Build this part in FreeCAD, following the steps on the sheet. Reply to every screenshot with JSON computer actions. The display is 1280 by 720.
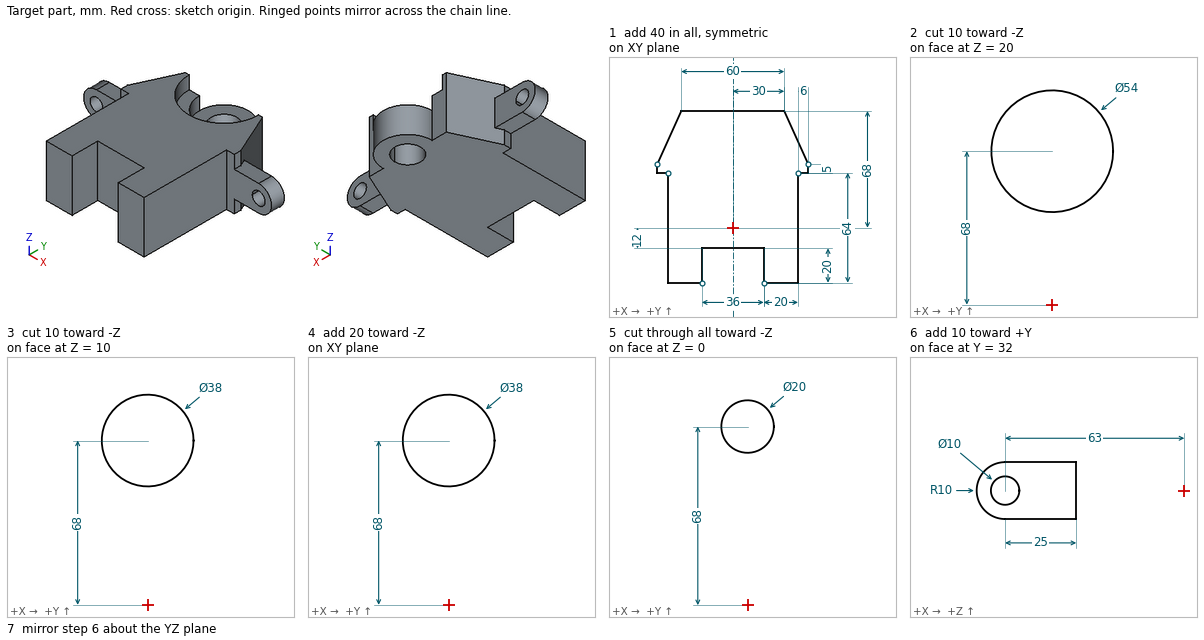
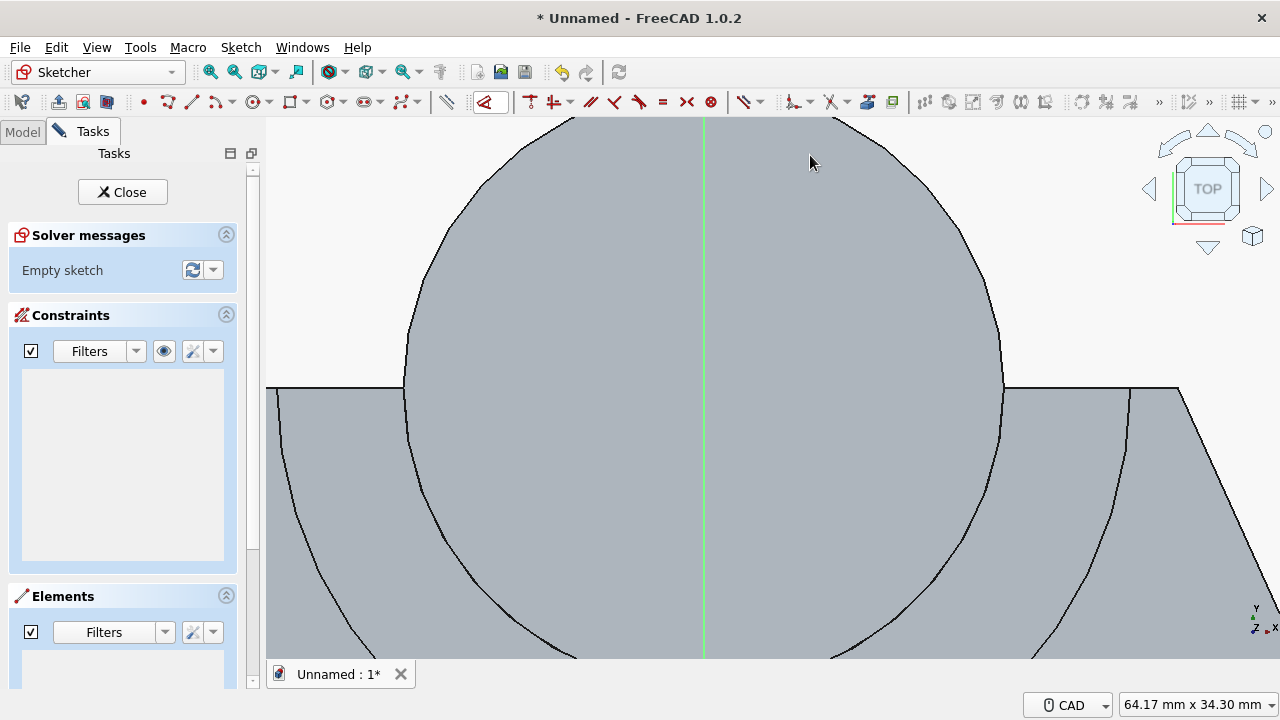
{"action": "left_click", "coordinate": [254, 102]}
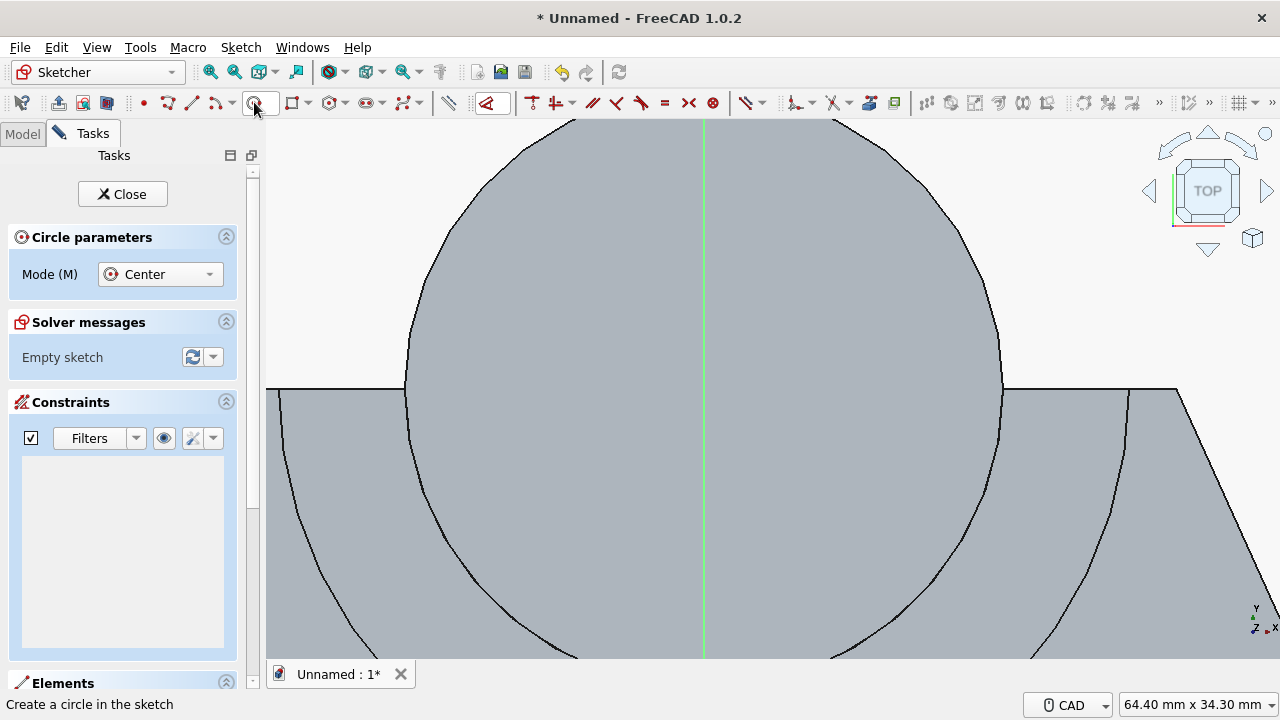
{"action": "left_click", "coordinate": [704, 389]}
{"action": "left_click", "coordinate": [815, 278]}
{"action": "key", "text": "Escape"}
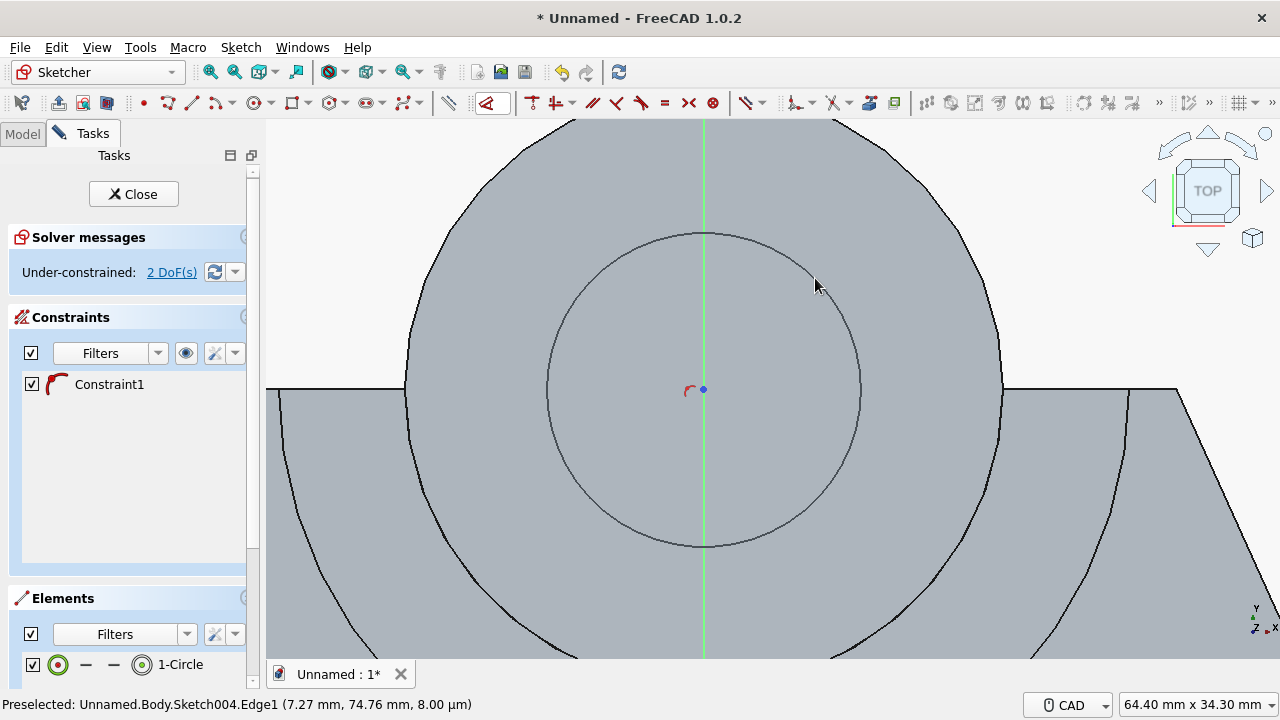
{"action": "left_click", "coordinate": [815, 279]}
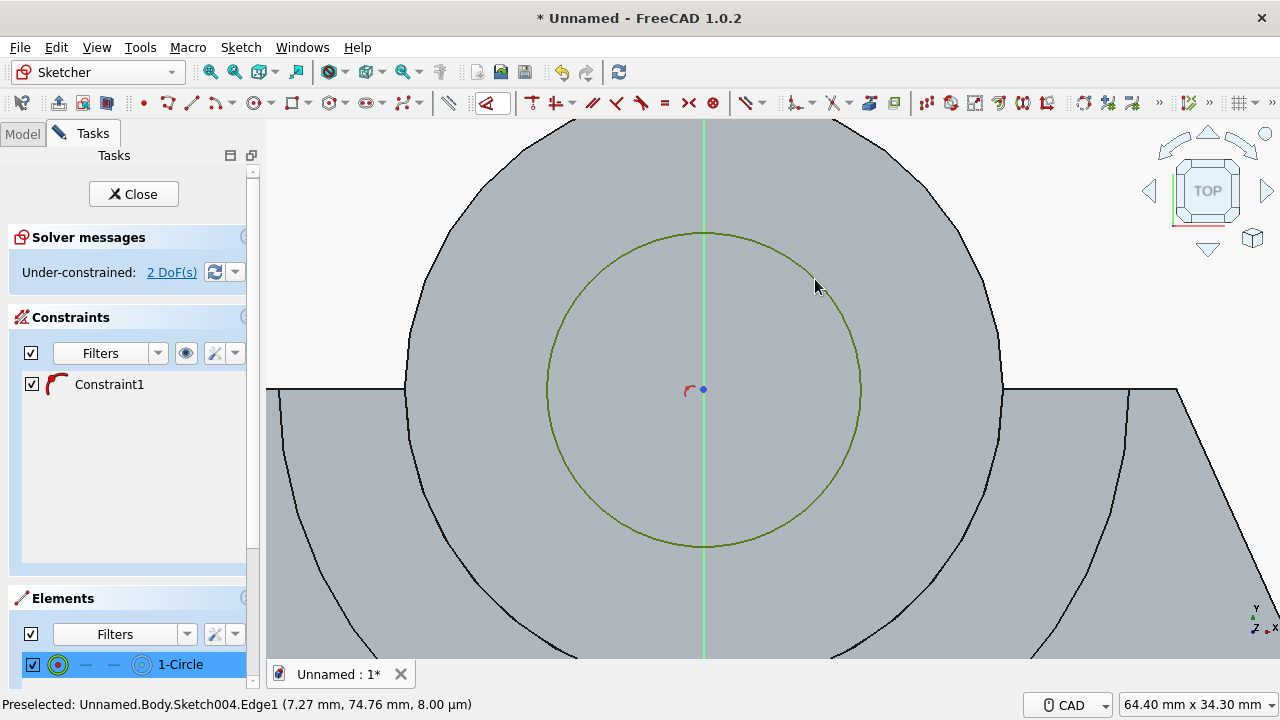
{"action": "key", "text": "k o"}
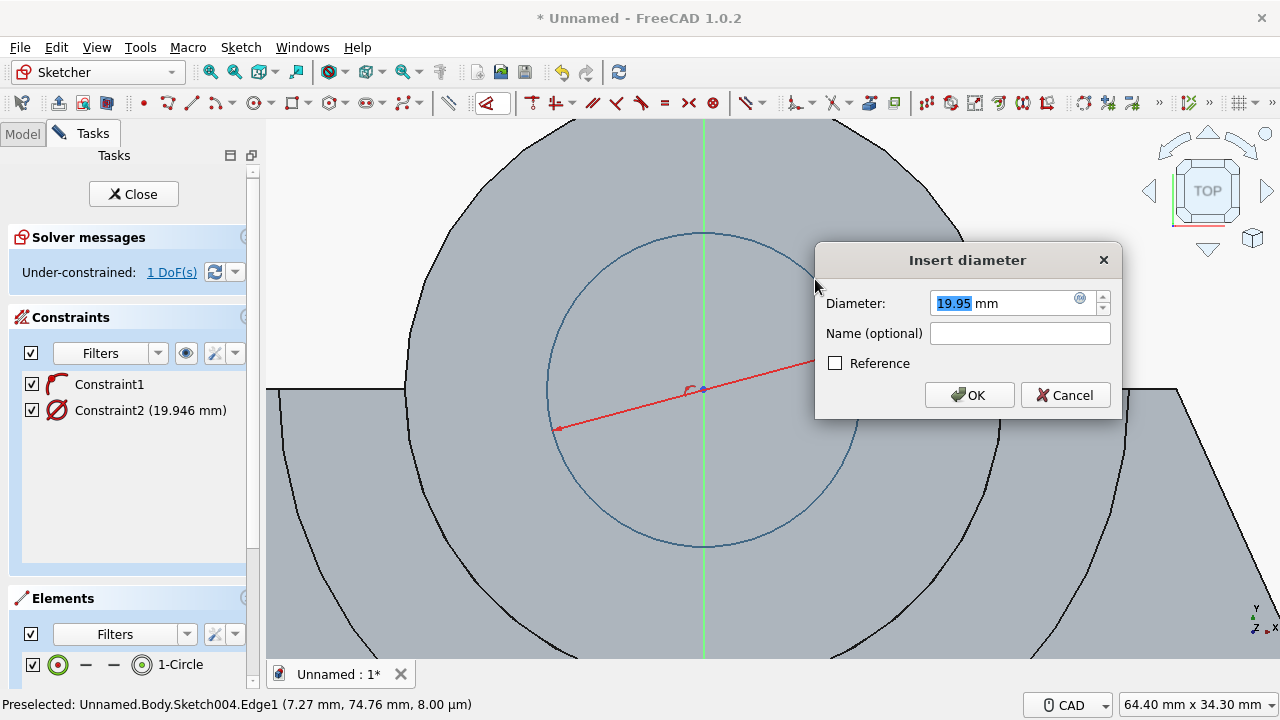
{"action": "type", "text": "20"}
{"action": "key", "text": "Return"}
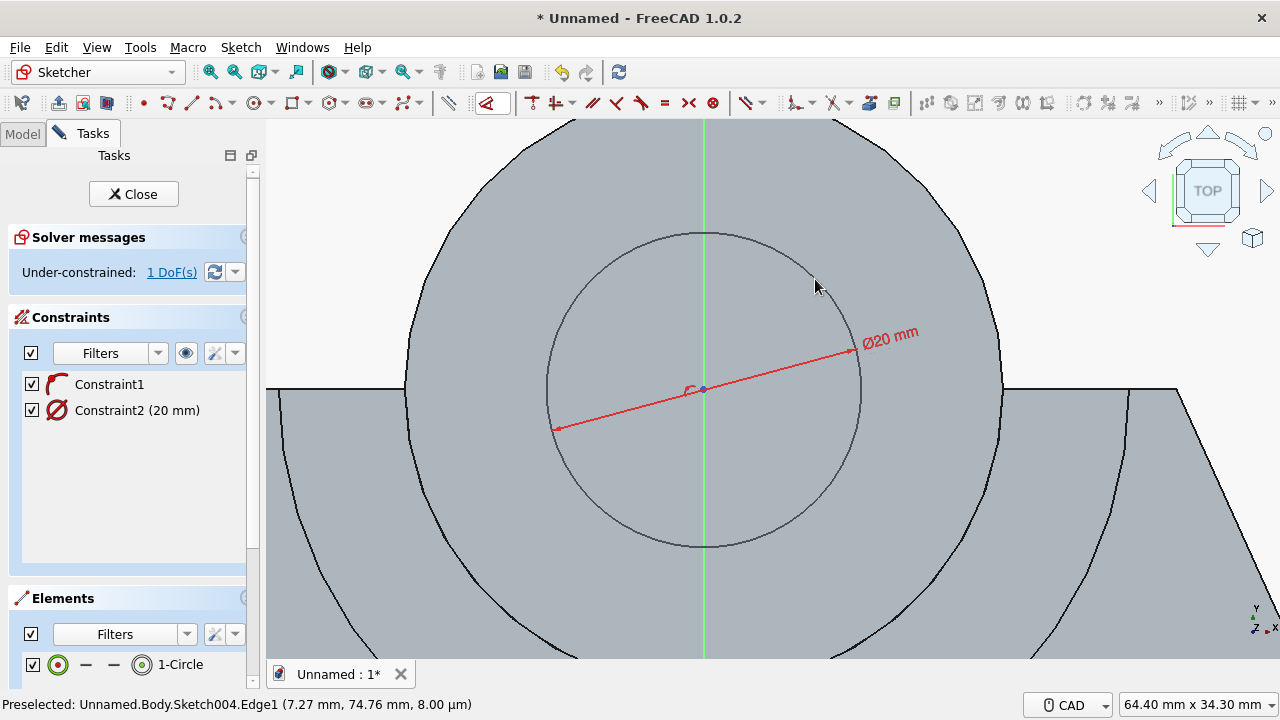
{"action": "left_click", "coordinate": [704, 390]}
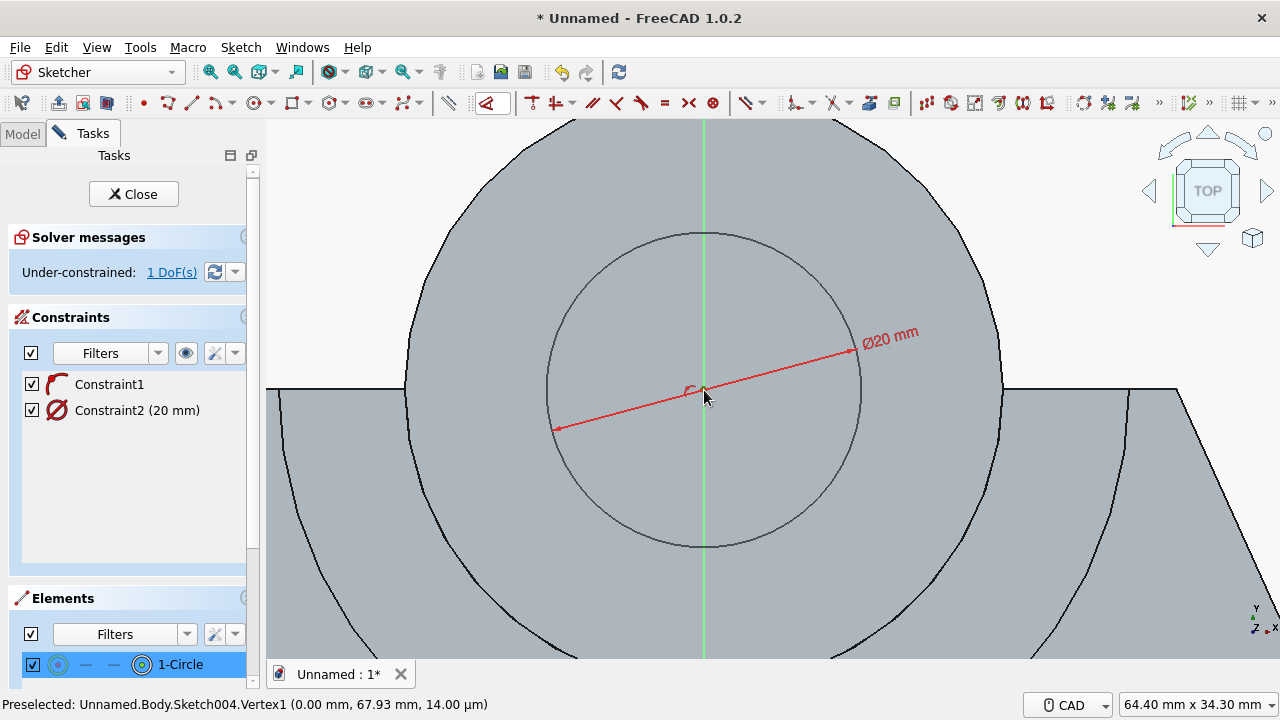
{"action": "left_click", "coordinate": [504, 104]}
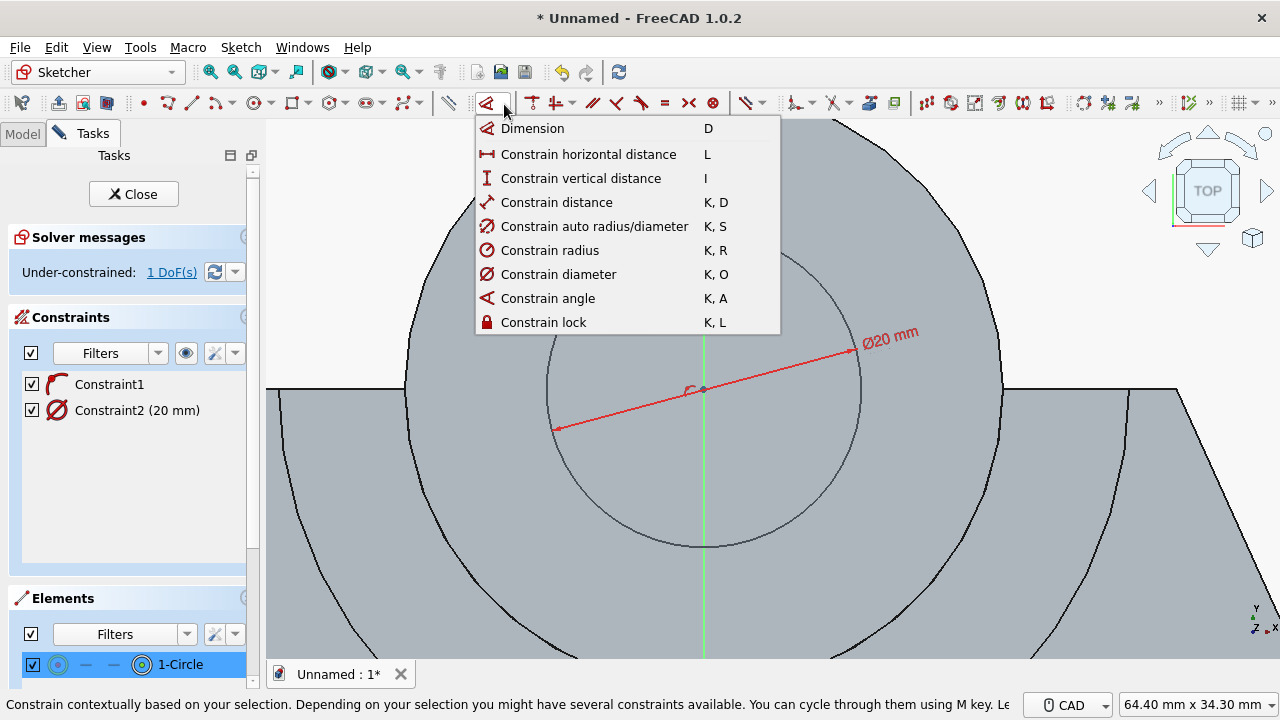
{"action": "left_click", "coordinate": [628, 178]}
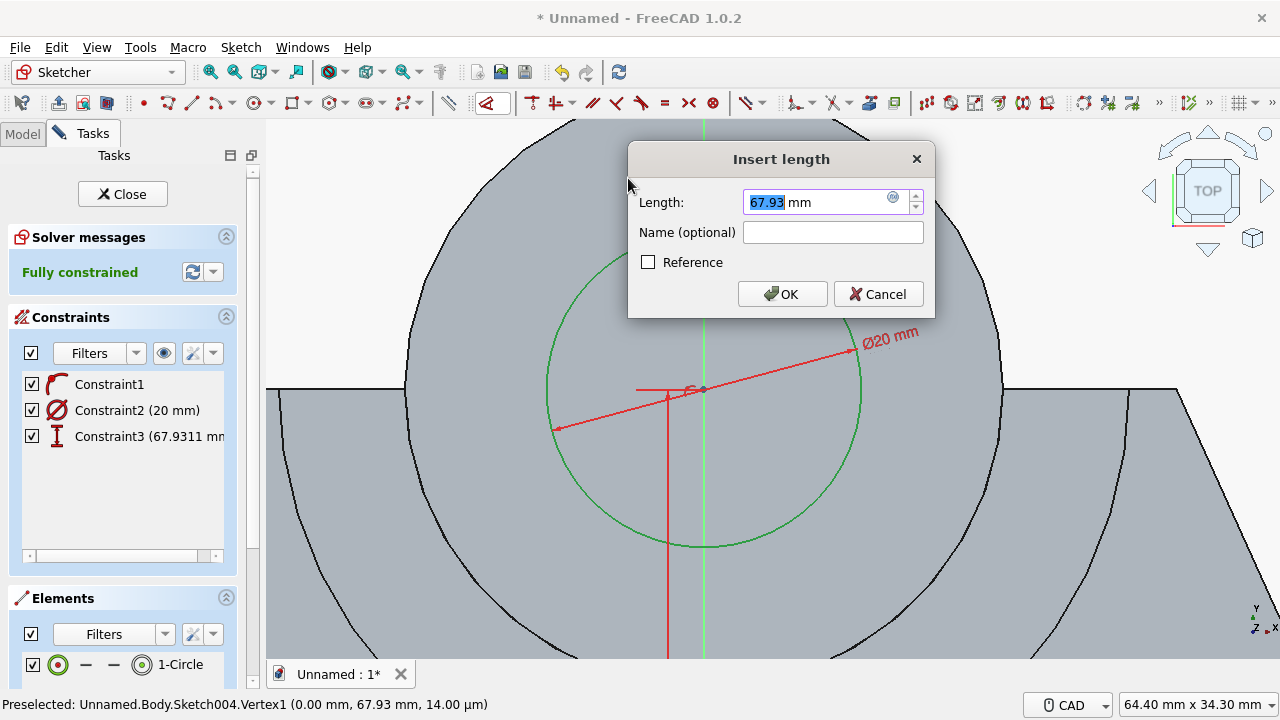
{"action": "type", "text": "68"}
{"action": "key", "text": "Return"}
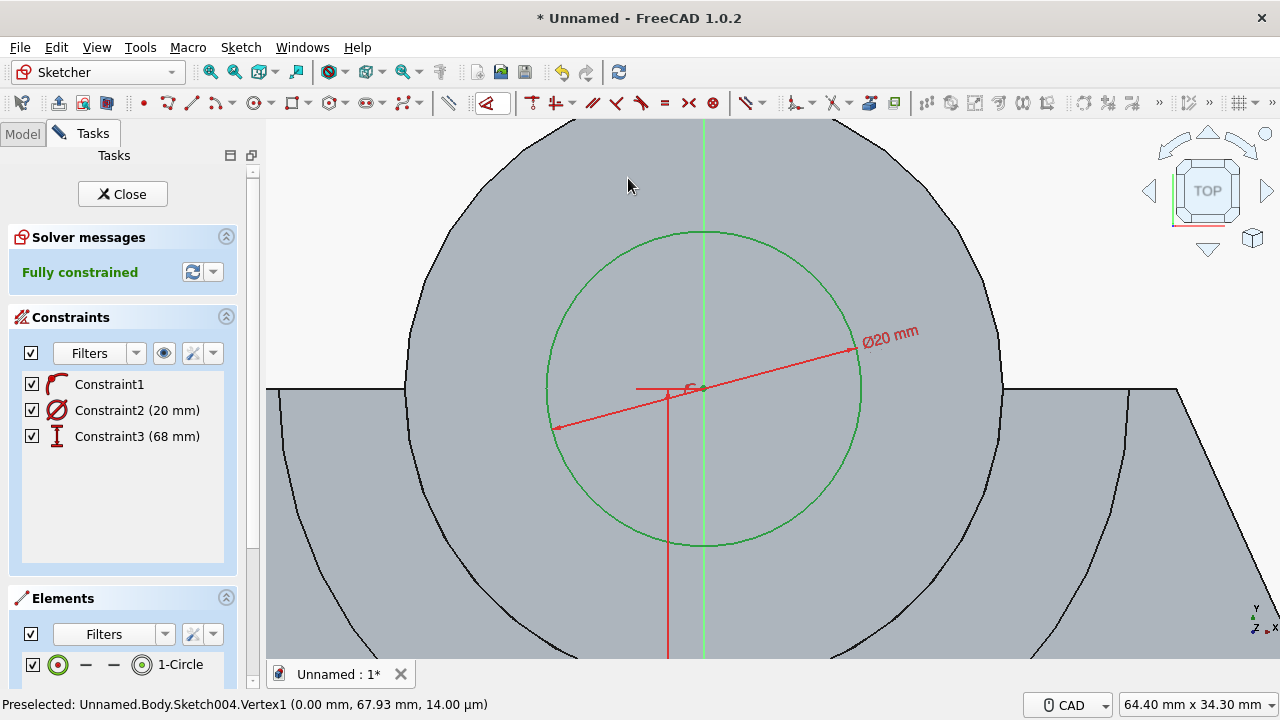
{"action": "left_click", "coordinate": [123, 194]}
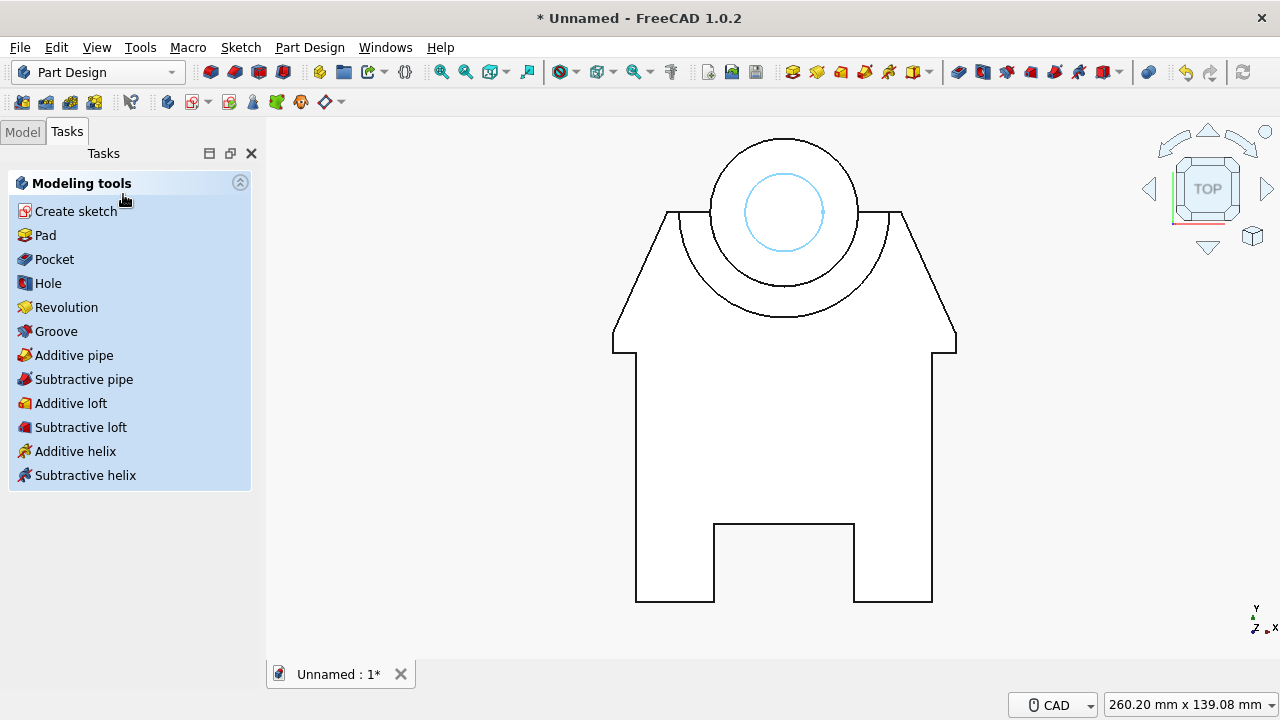
{"action": "left_click", "coordinate": [960, 72]}